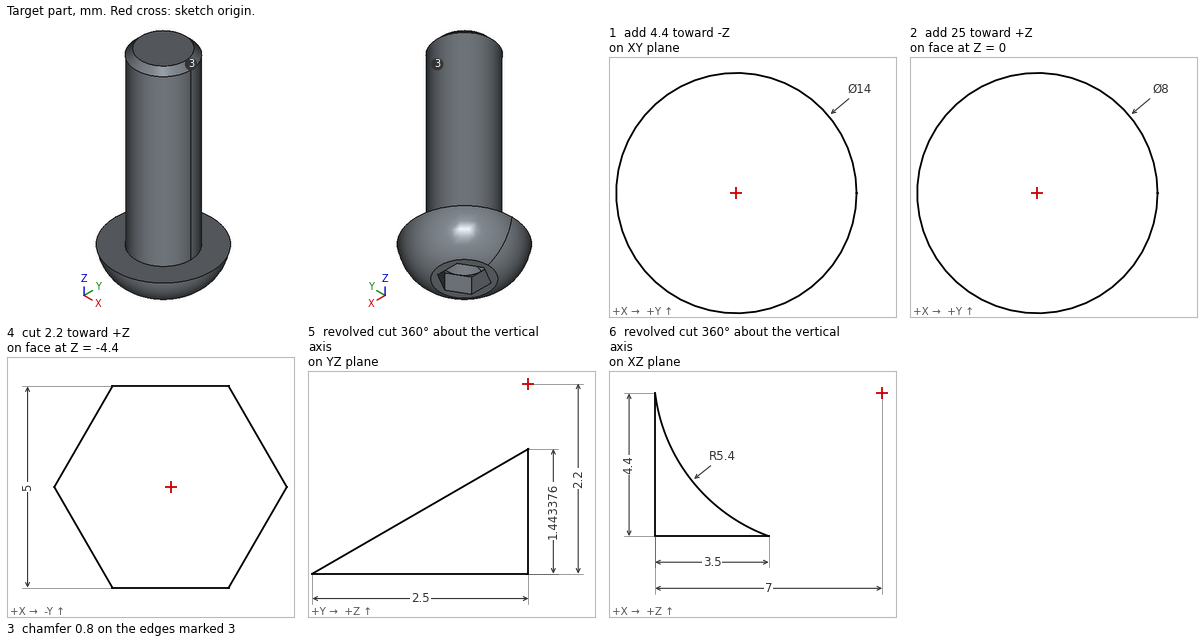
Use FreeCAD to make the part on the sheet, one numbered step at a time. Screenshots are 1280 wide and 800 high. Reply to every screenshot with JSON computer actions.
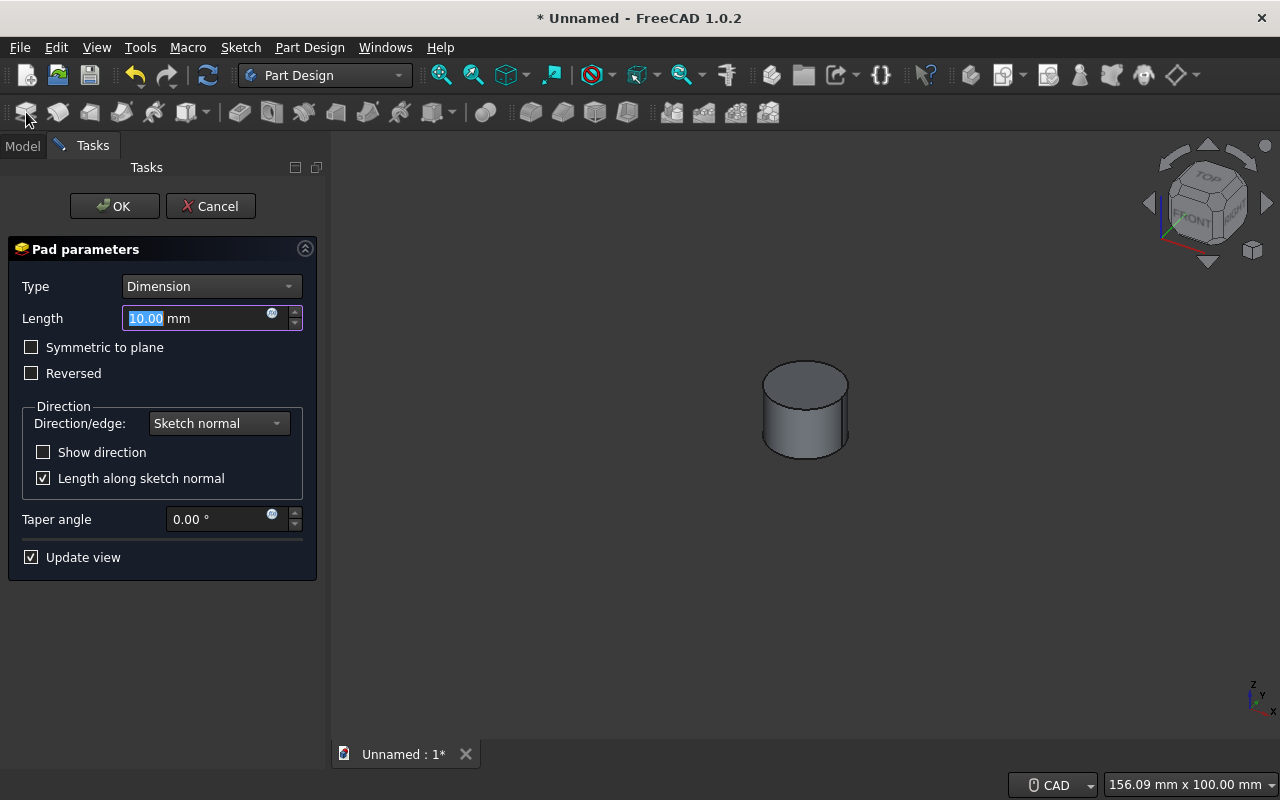
{"action": "type", "text": "4.4"}
{"action": "key", "text": "Tab"}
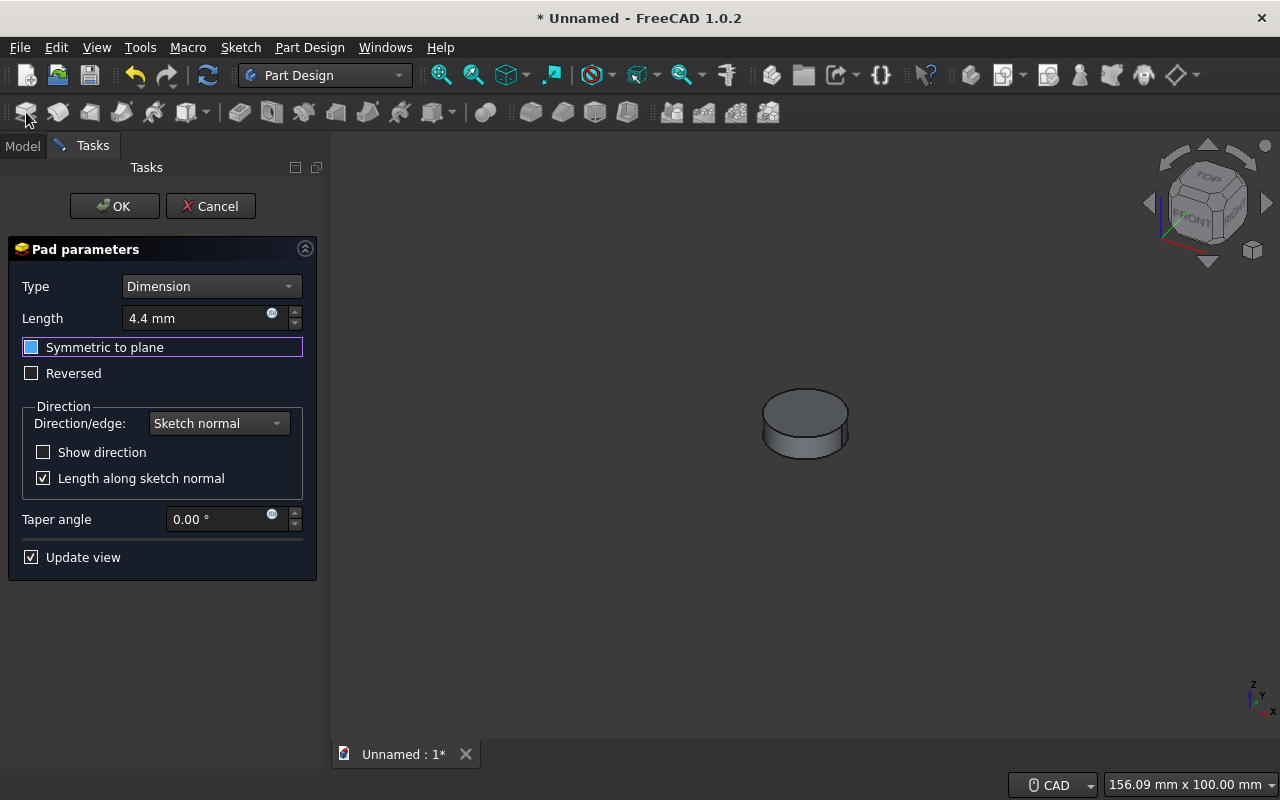
{"action": "left_click", "coordinate": [30, 373]}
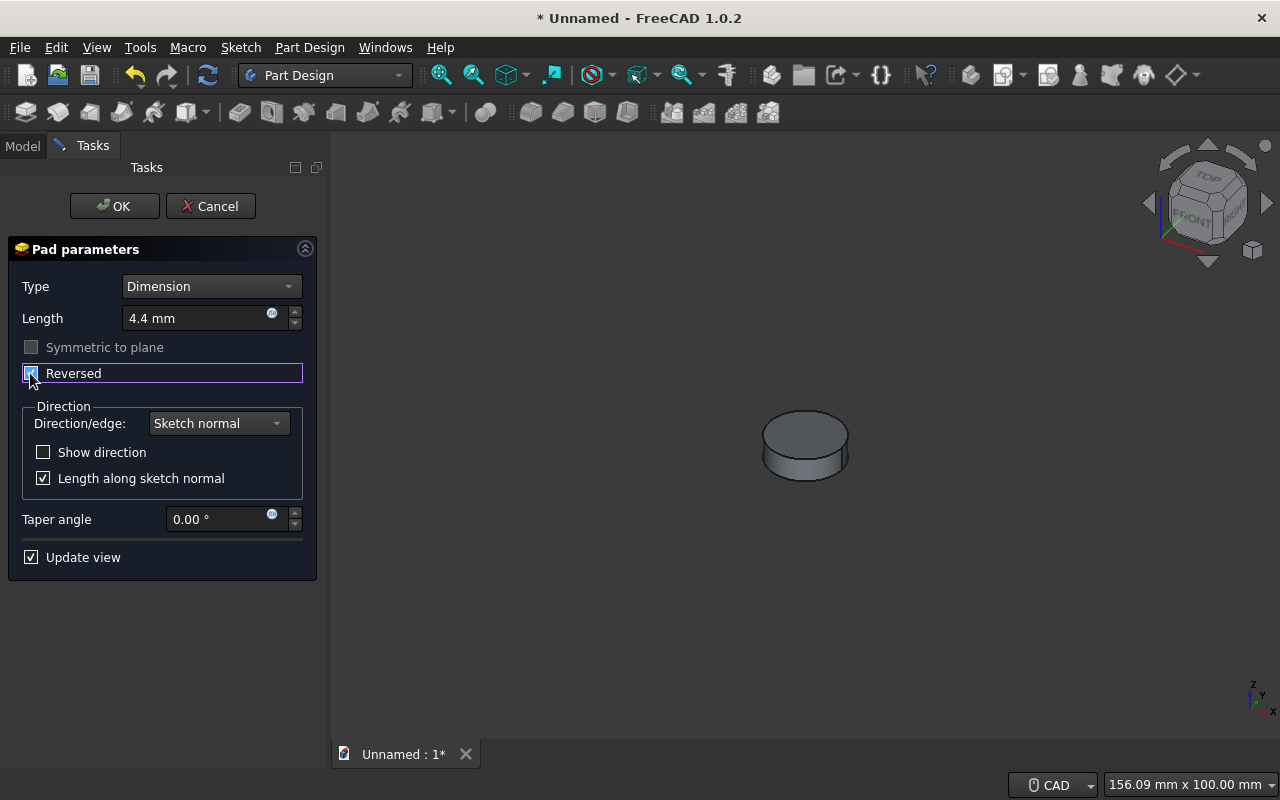
{"action": "left_click", "coordinate": [115, 206]}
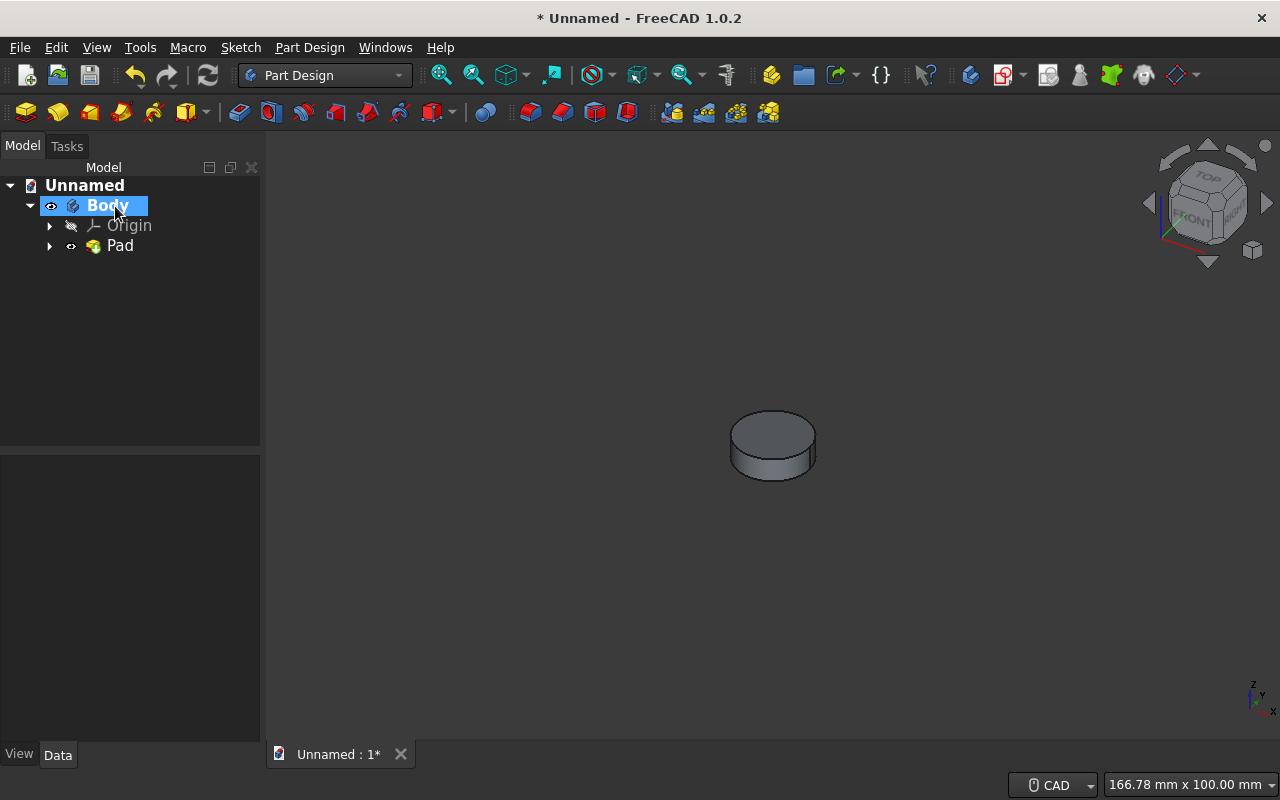
{"action": "key", "text": "v f"}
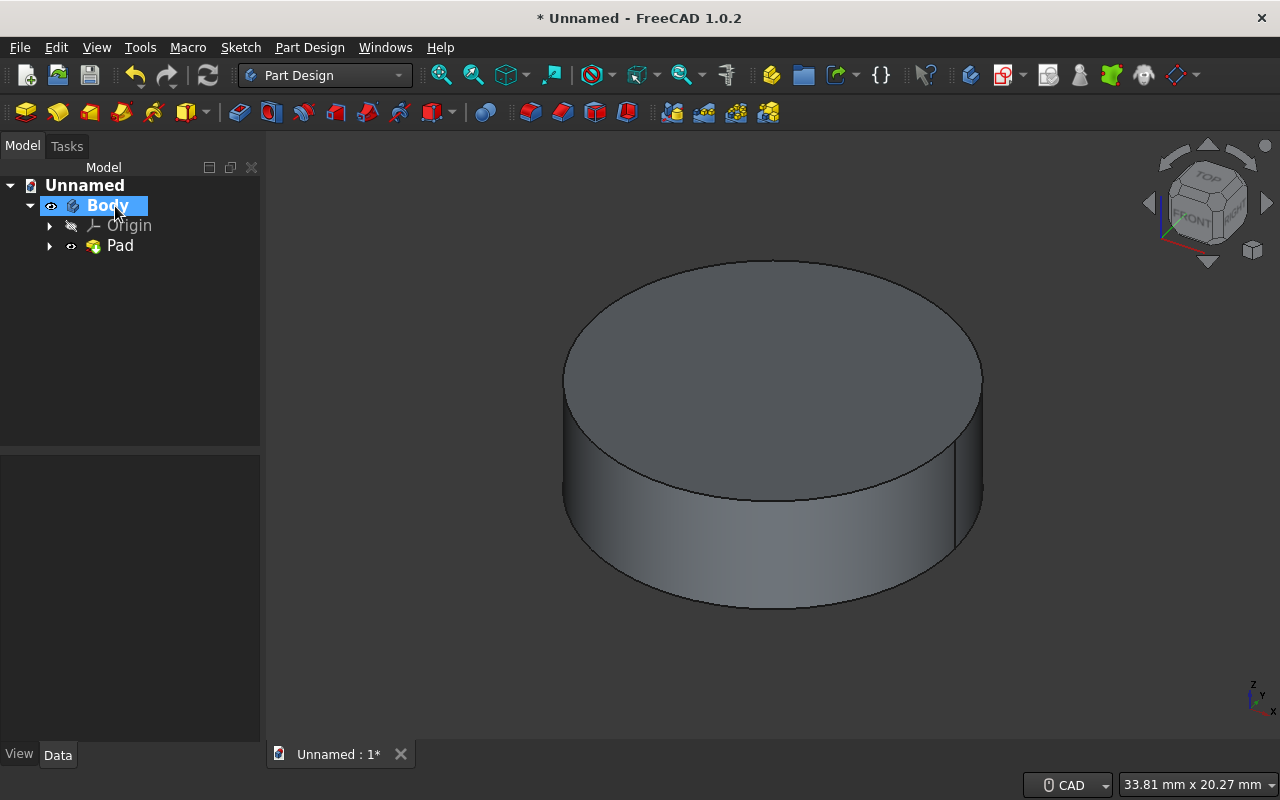
{"action": "left_click", "coordinate": [773, 380]}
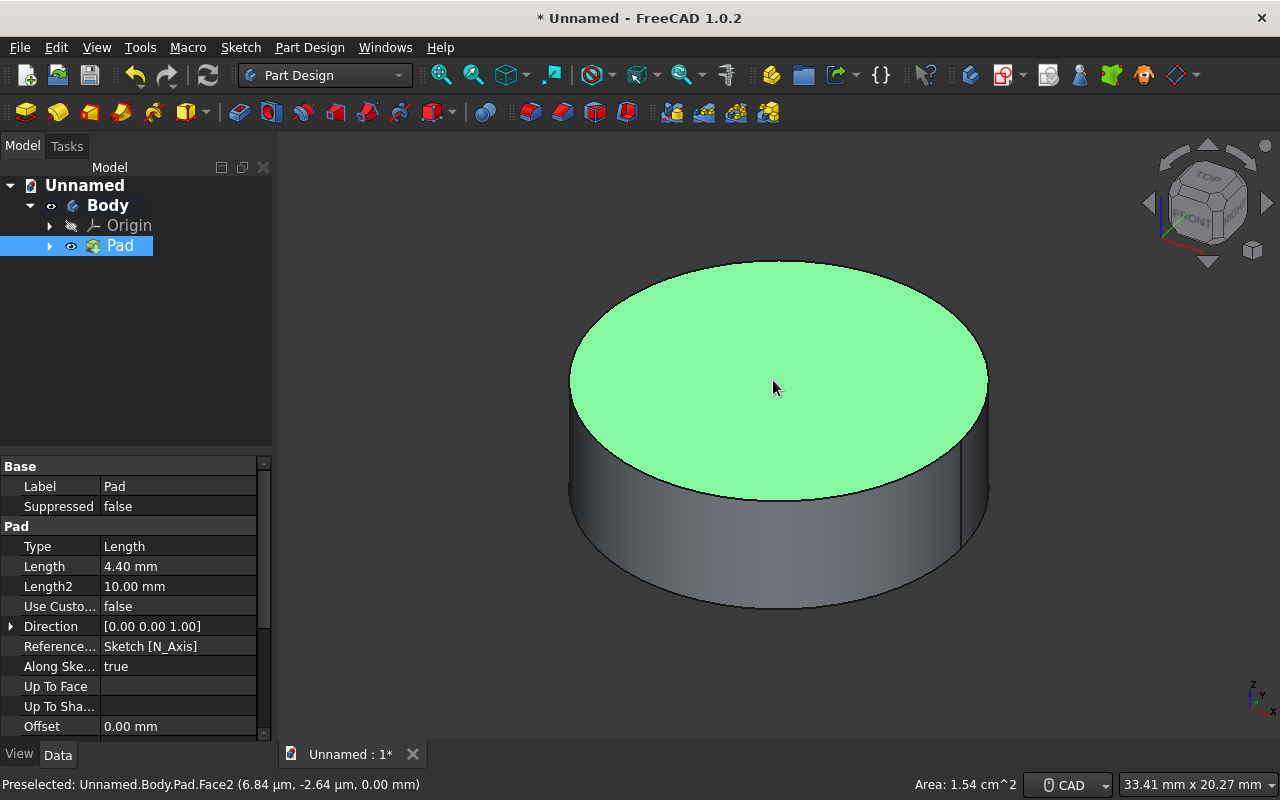
{"action": "left_click", "coordinate": [1004, 76]}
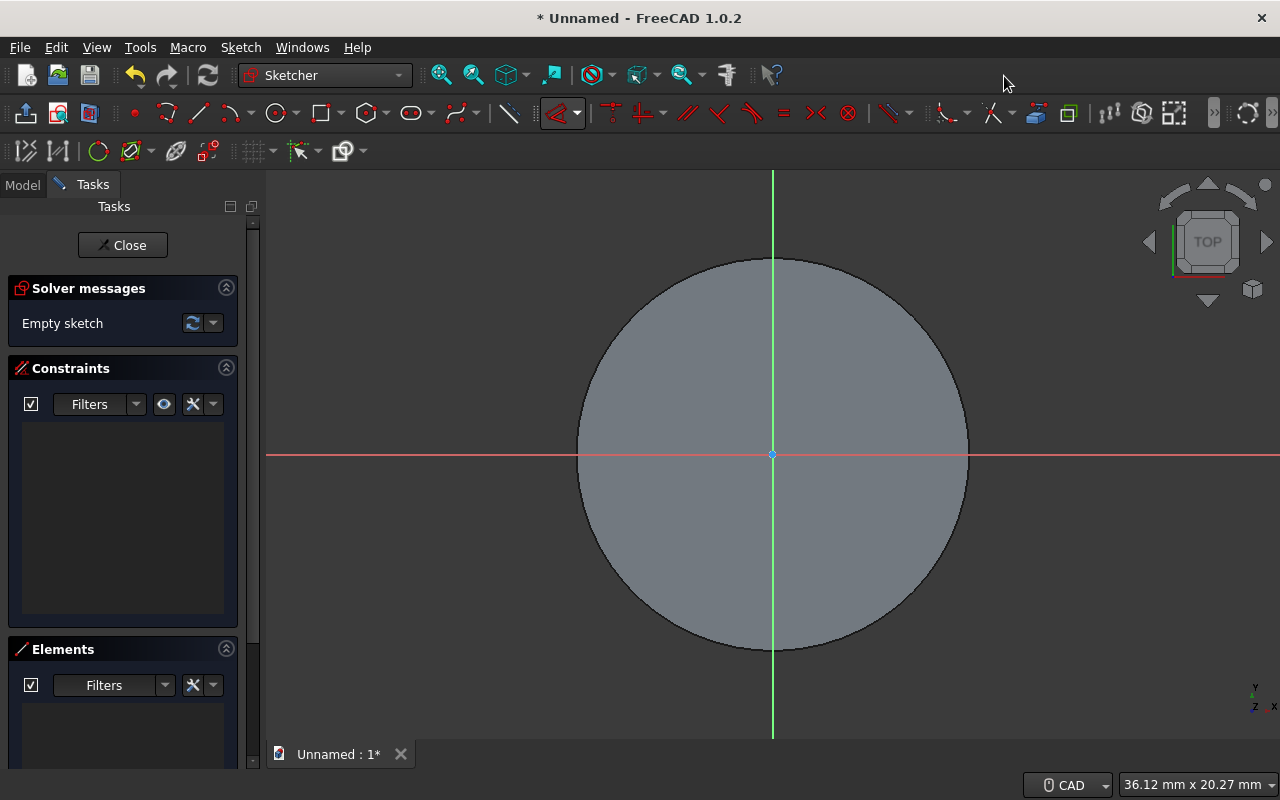
{"action": "scroll", "coordinate": [912, 455], "scroll_direction": "up", "scroll_amount": 2}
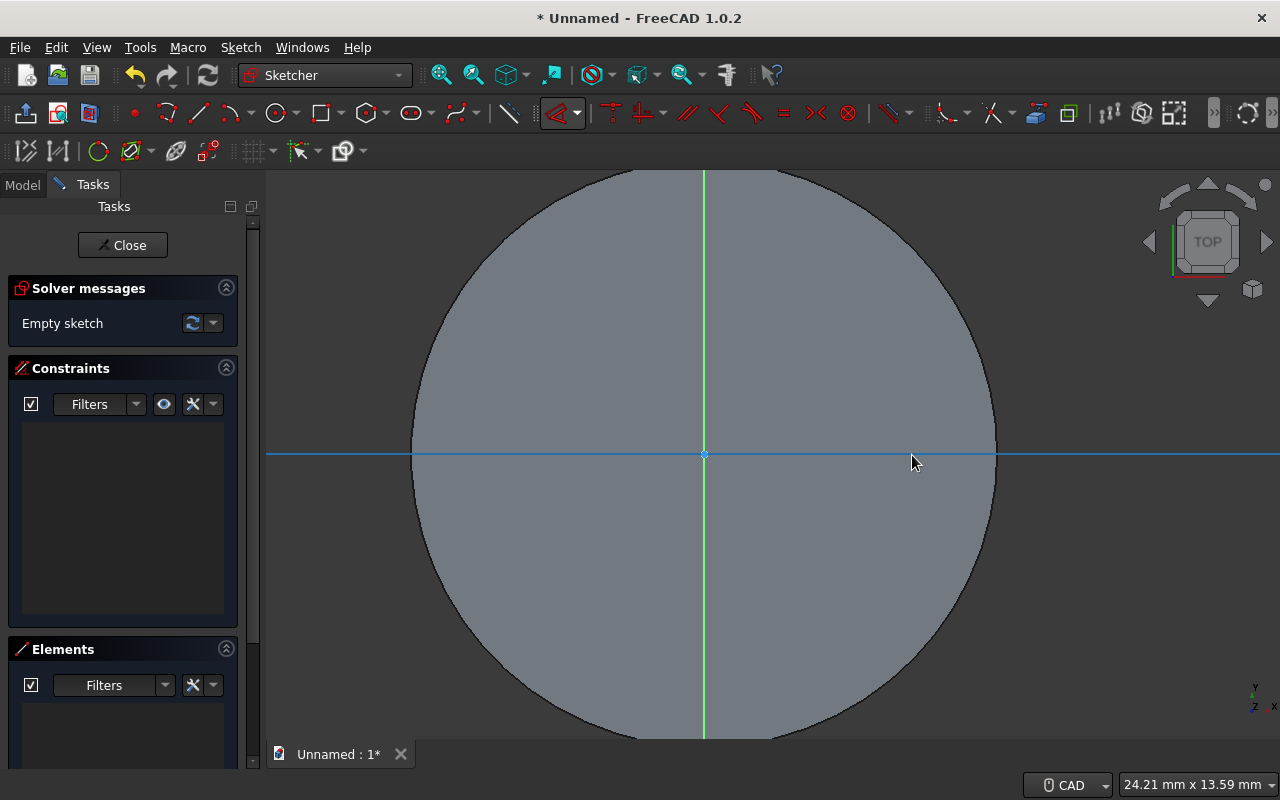
{"action": "left_click", "coordinate": [276, 114]}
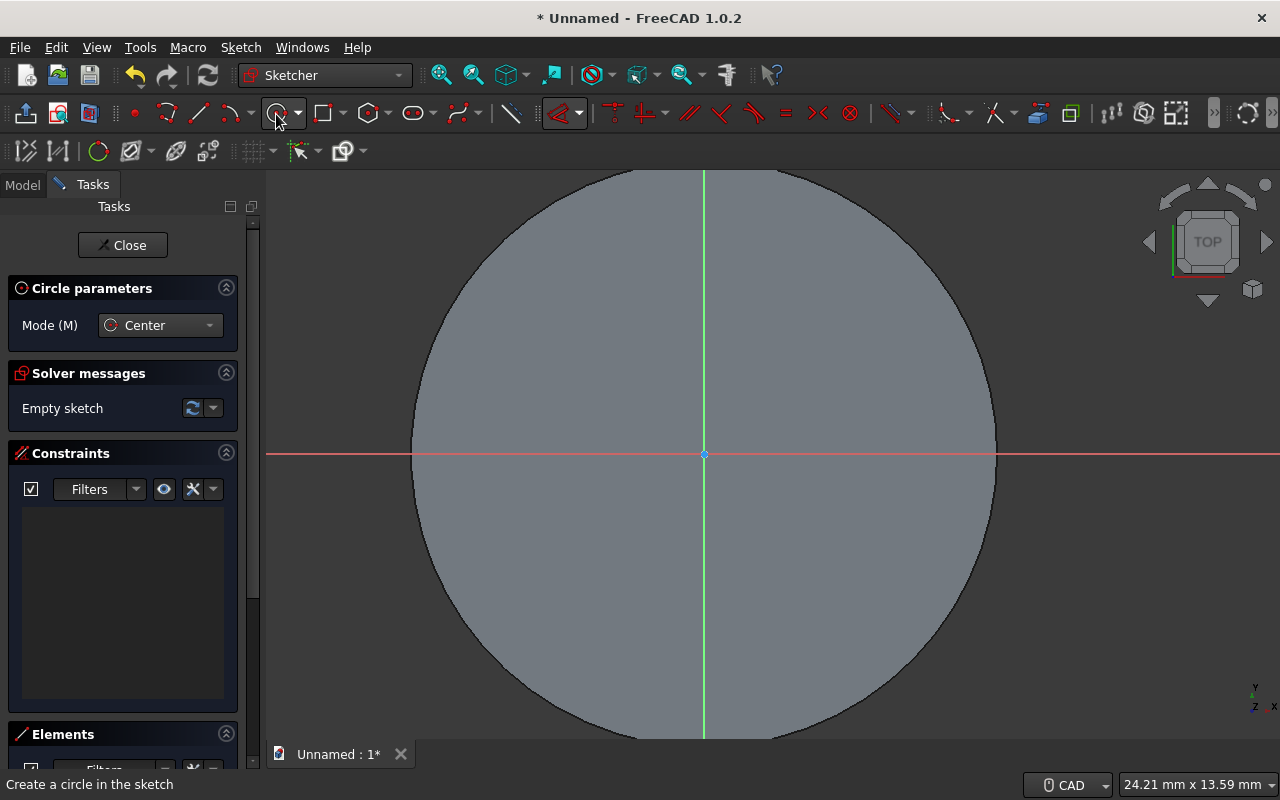
{"action": "left_click", "coordinate": [704, 454]}
{"action": "mouse_move", "coordinate": [823, 336]}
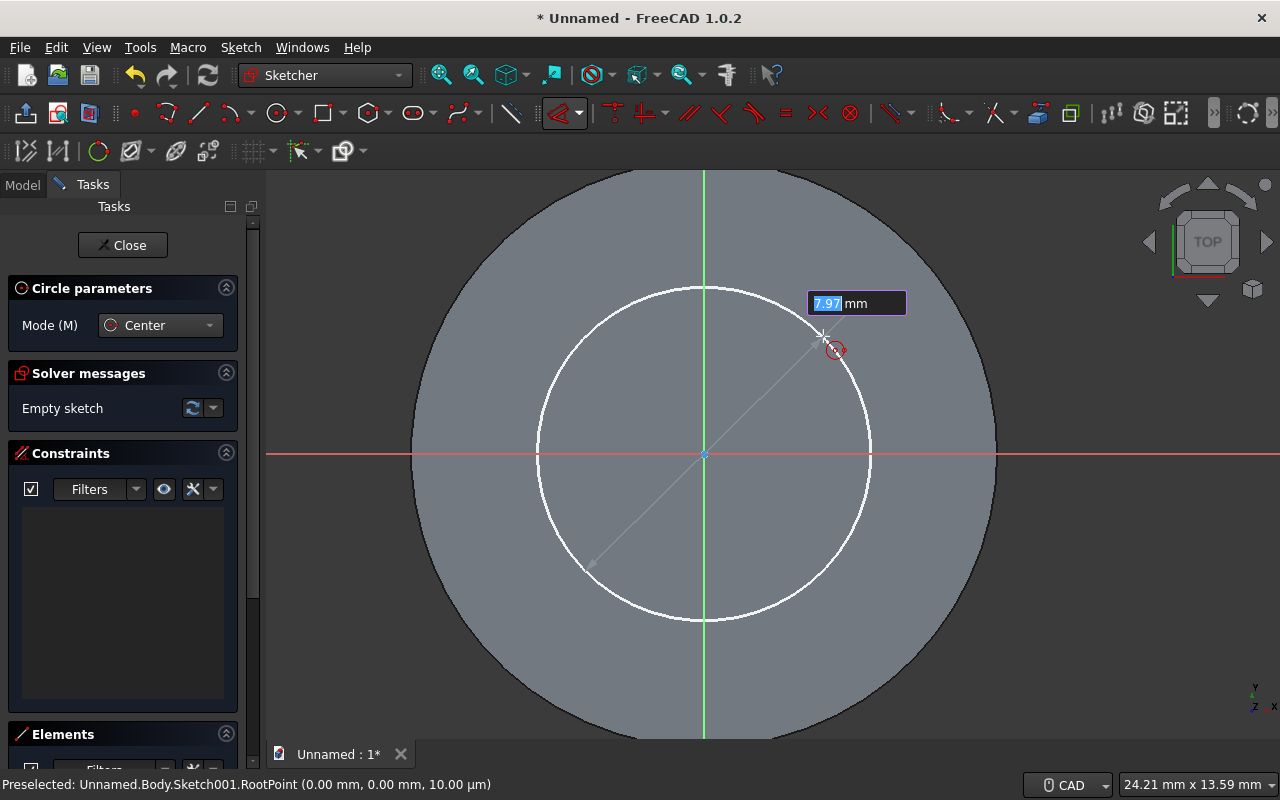
{"action": "type", "text": "8"}
{"action": "key", "text": "Return"}
{"action": "key", "text": "Escape"}